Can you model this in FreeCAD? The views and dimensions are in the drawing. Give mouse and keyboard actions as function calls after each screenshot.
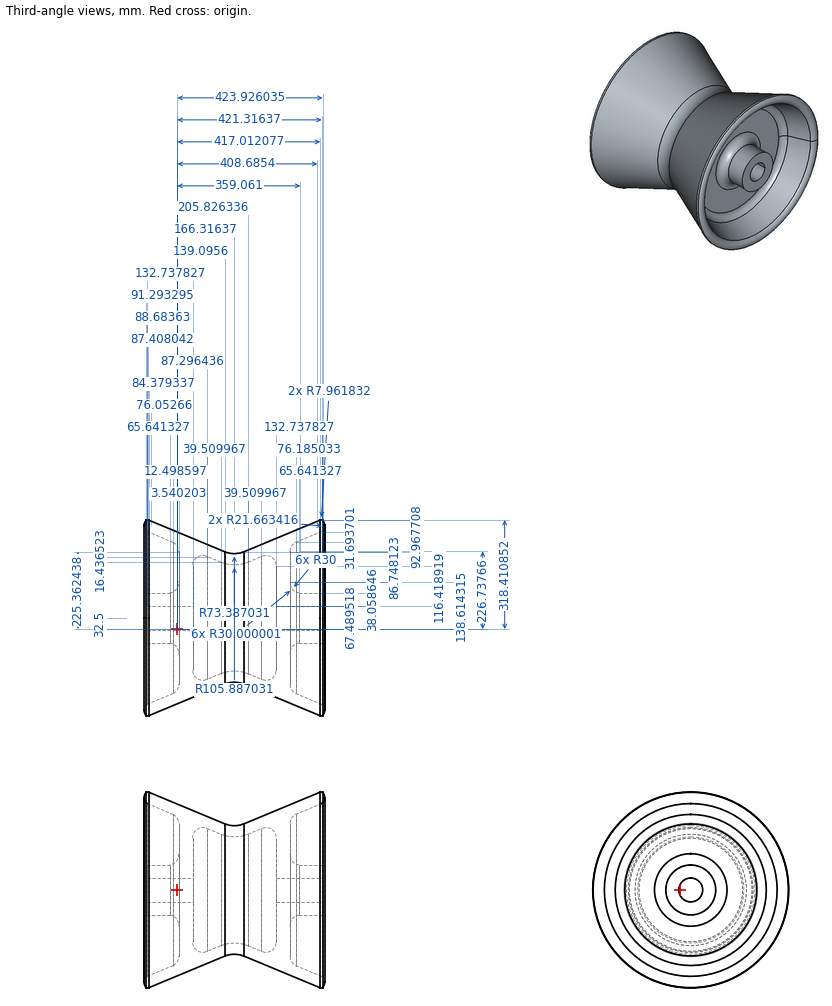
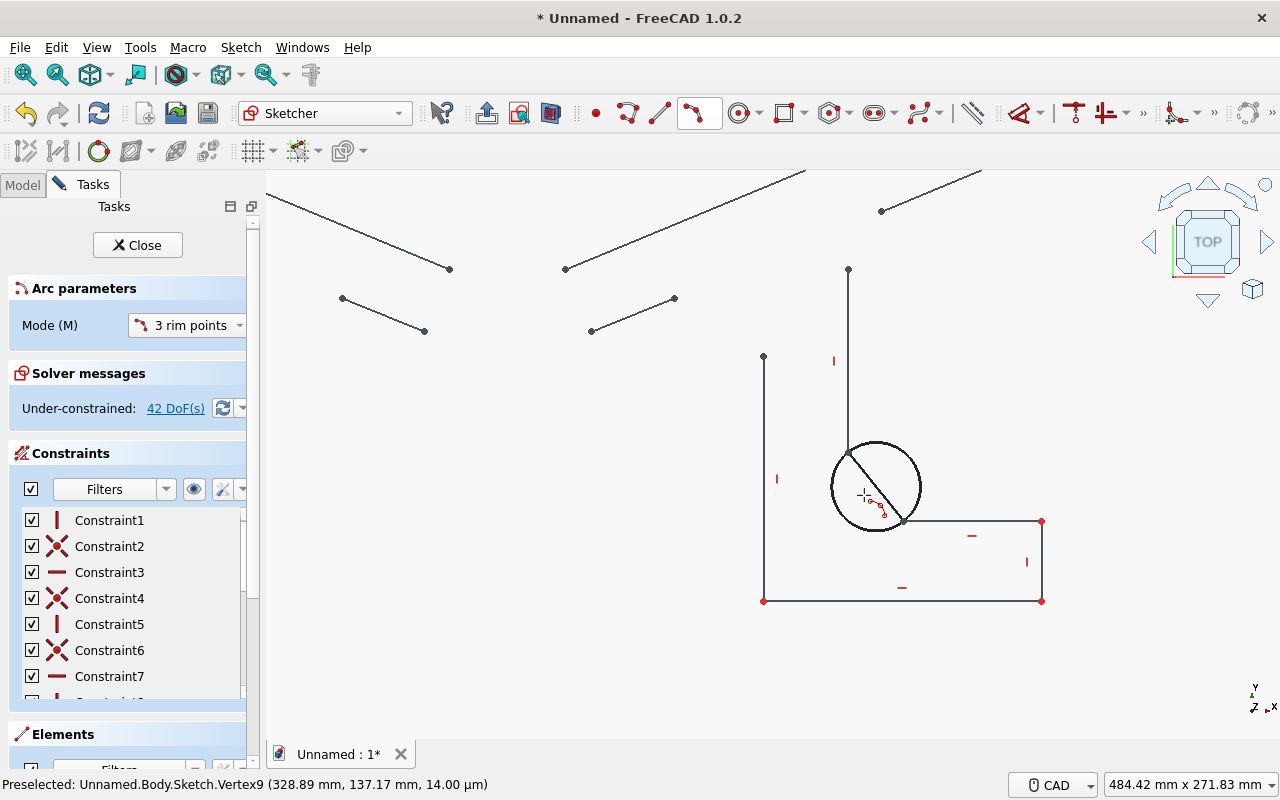
click(862, 495)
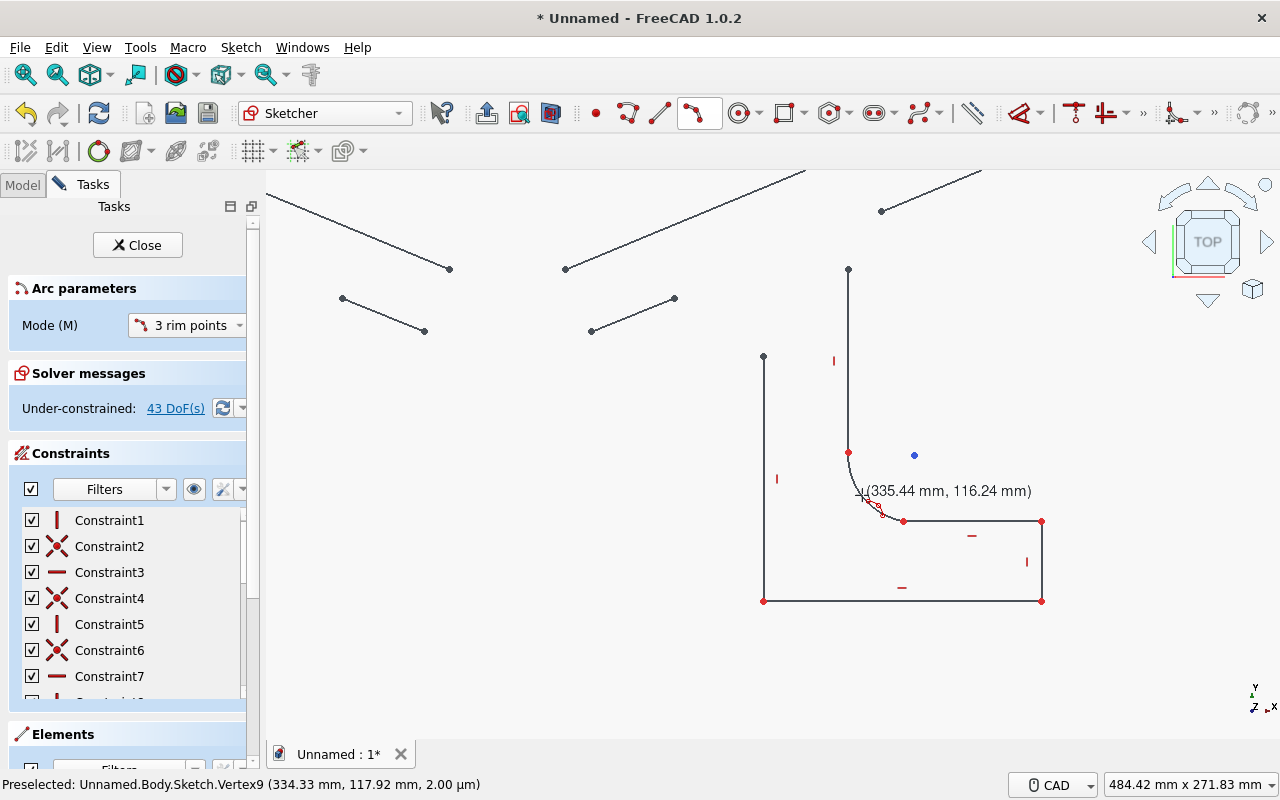
click(848, 270)
click(882, 212)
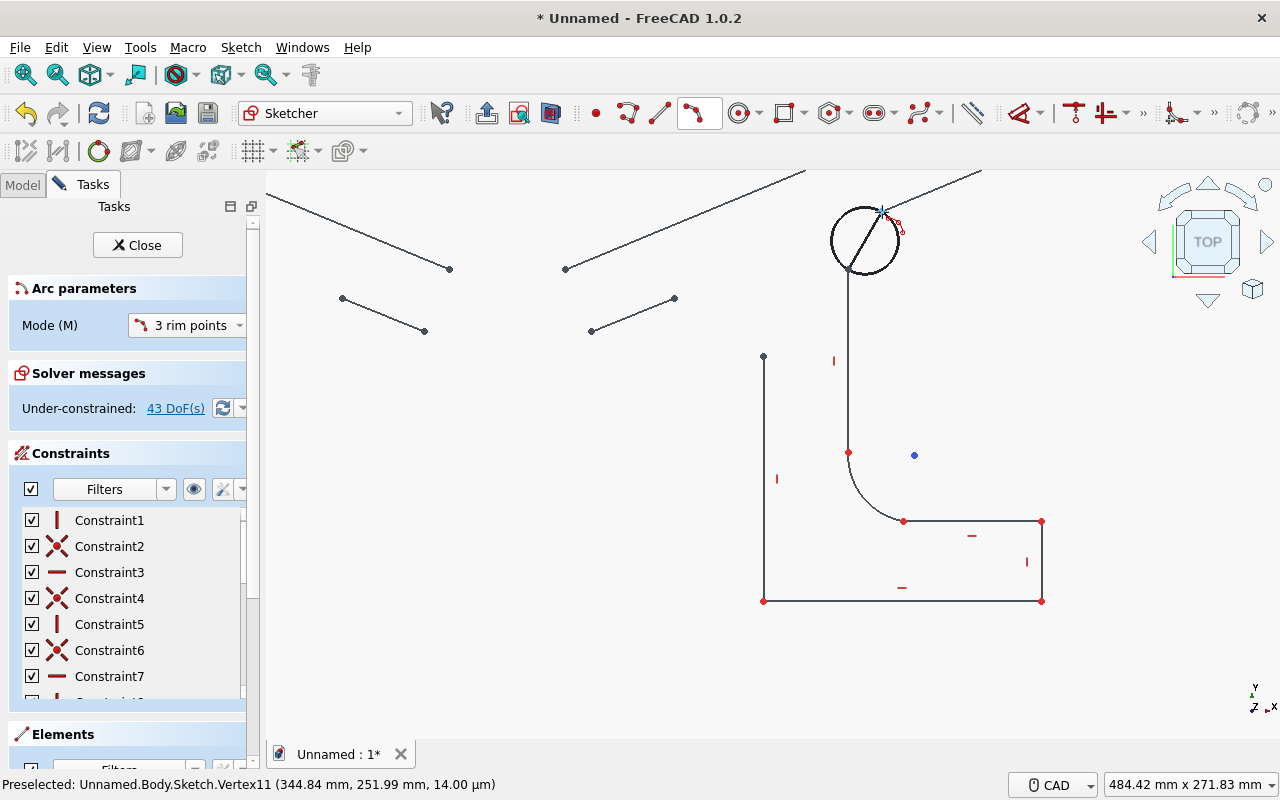
scroll(857, 233, up, 3)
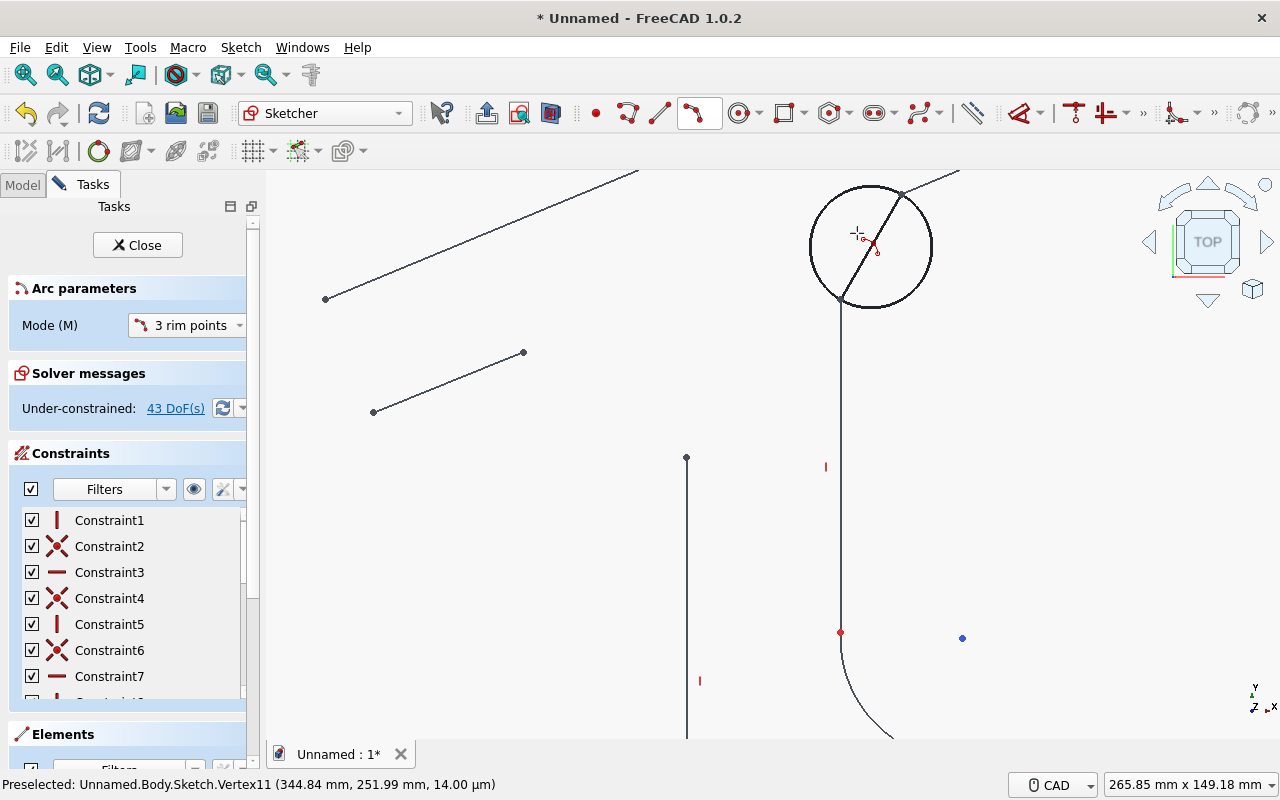
click(857, 234)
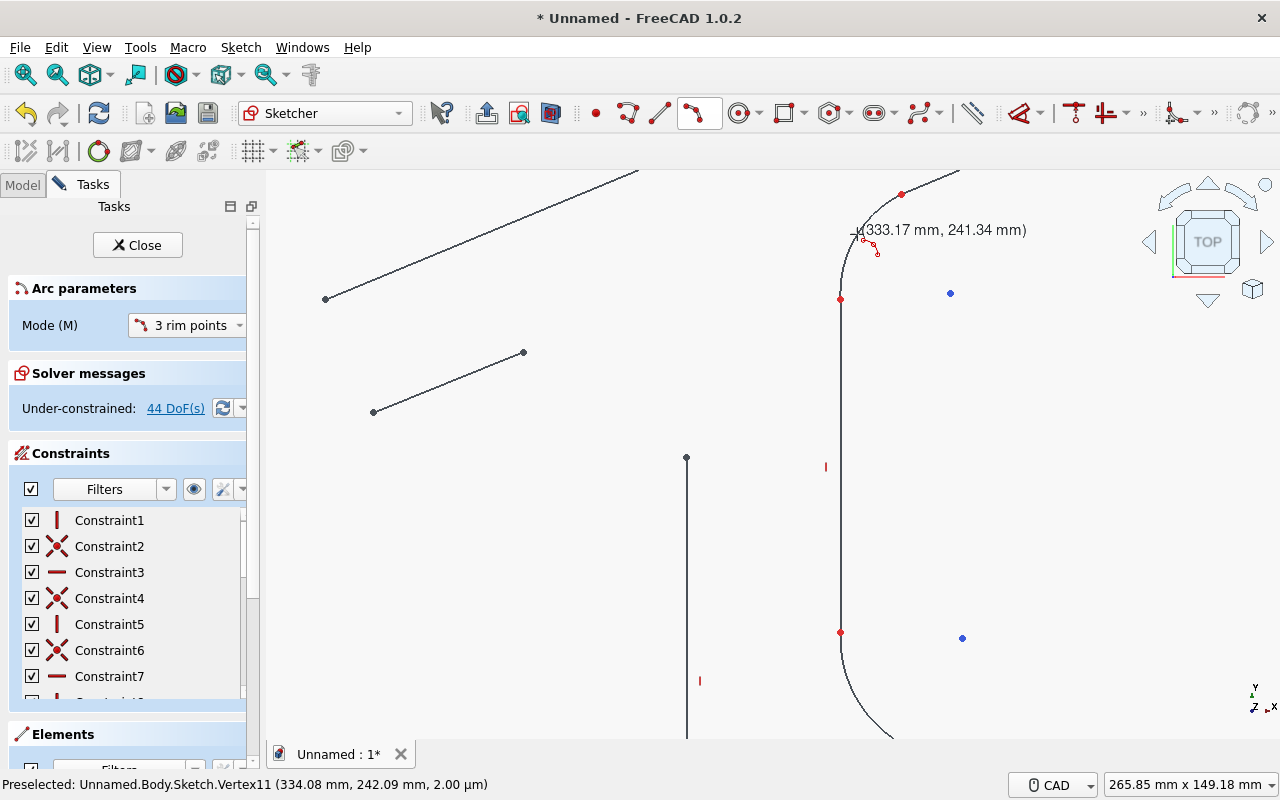
scroll(863, 424, down, 7)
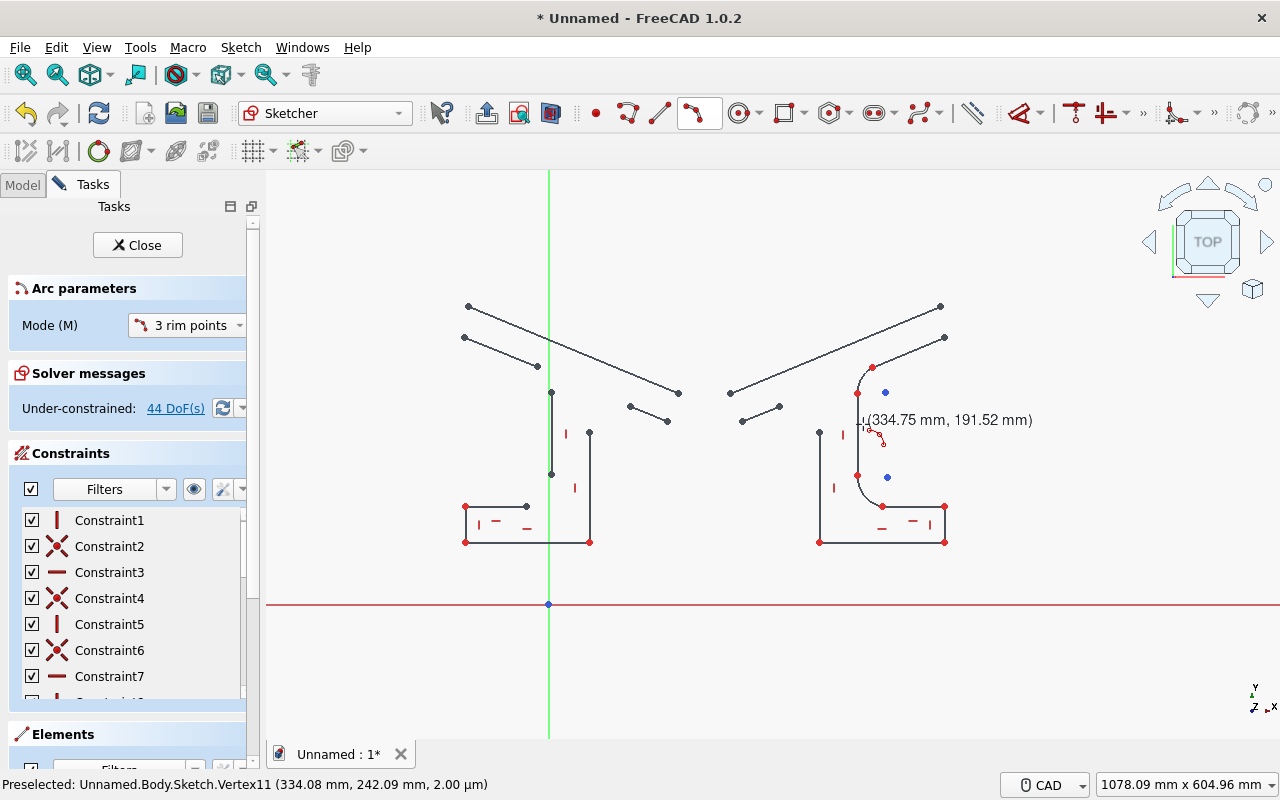
click(945, 338)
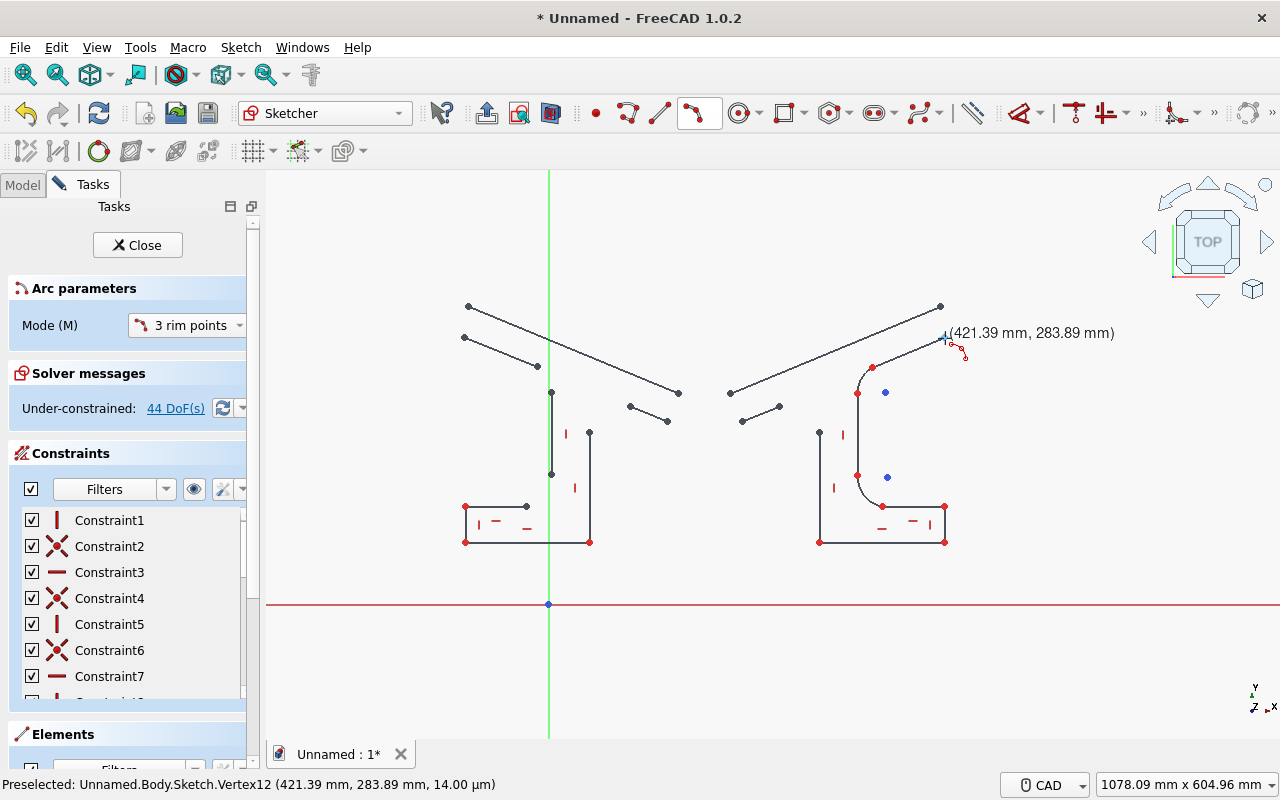
scroll(947, 306, up, 5)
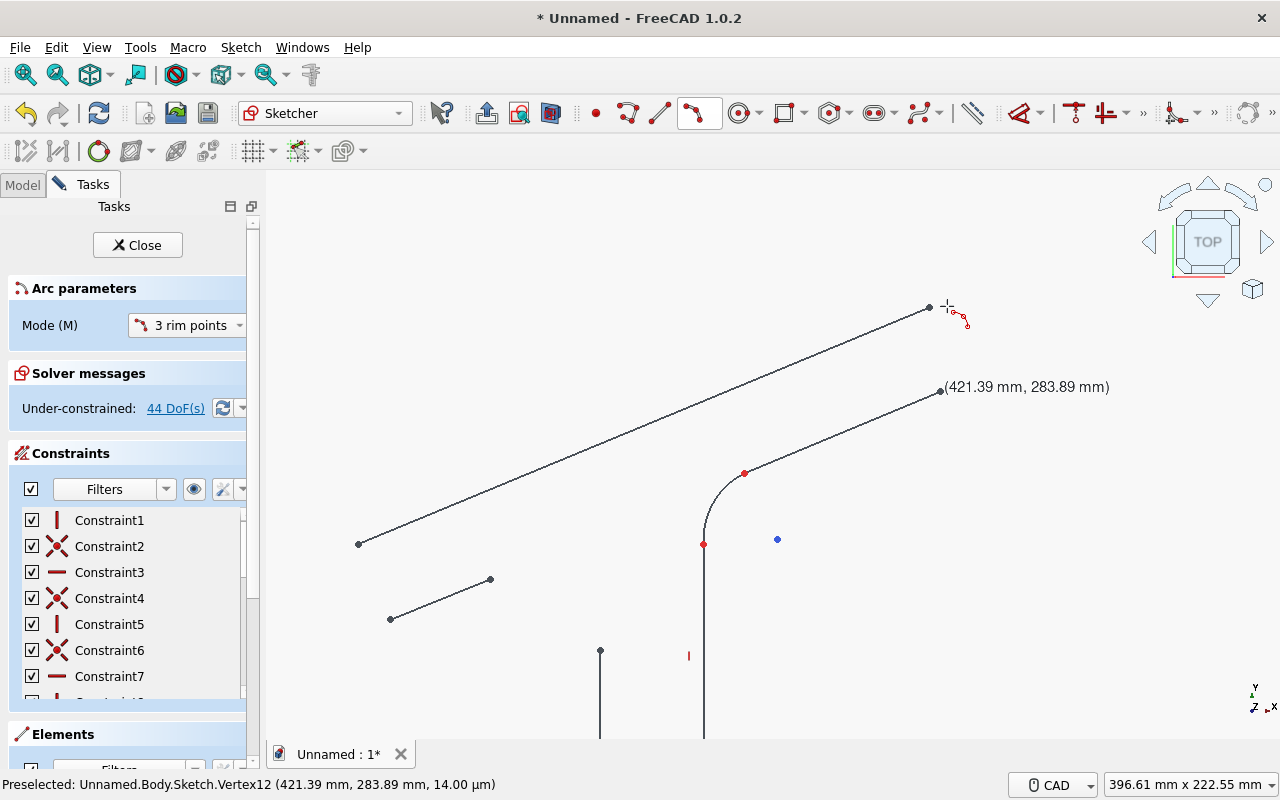
click(947, 305)
click(963, 348)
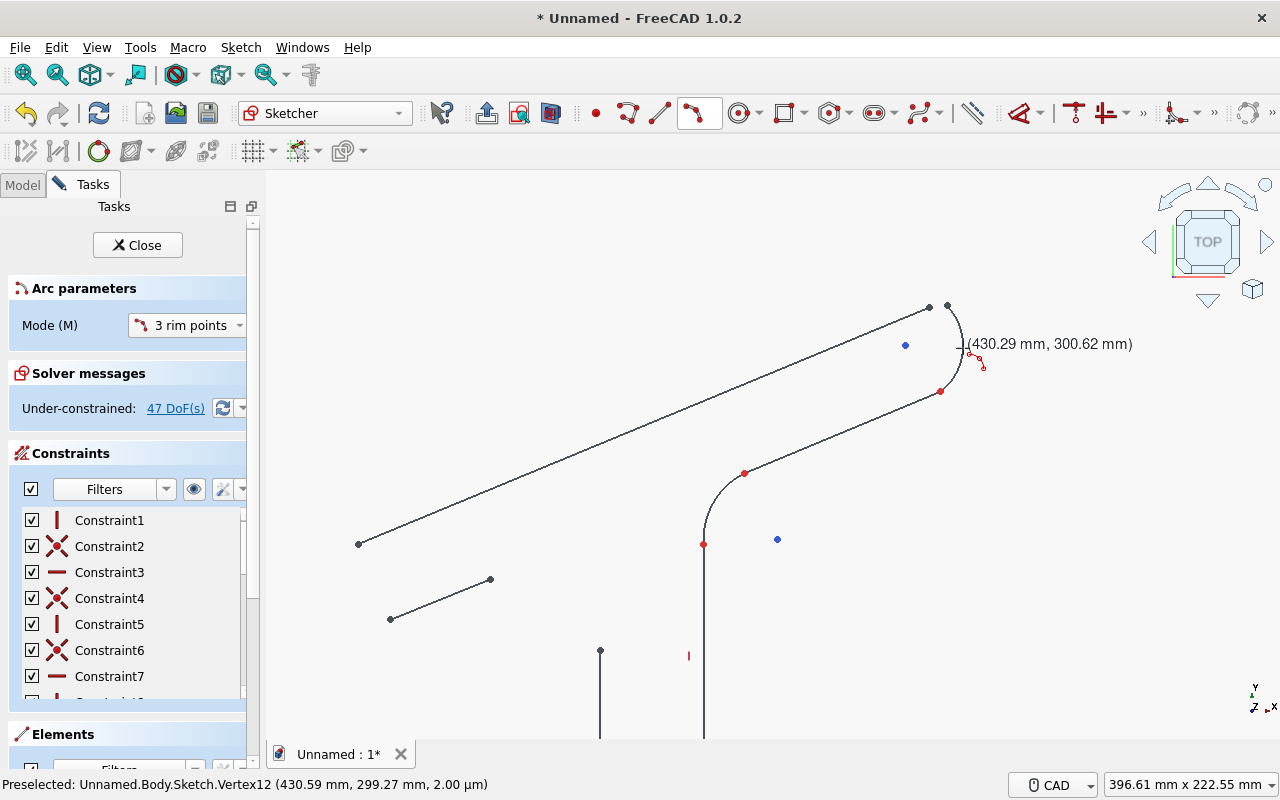
click(947, 306)
click(929, 308)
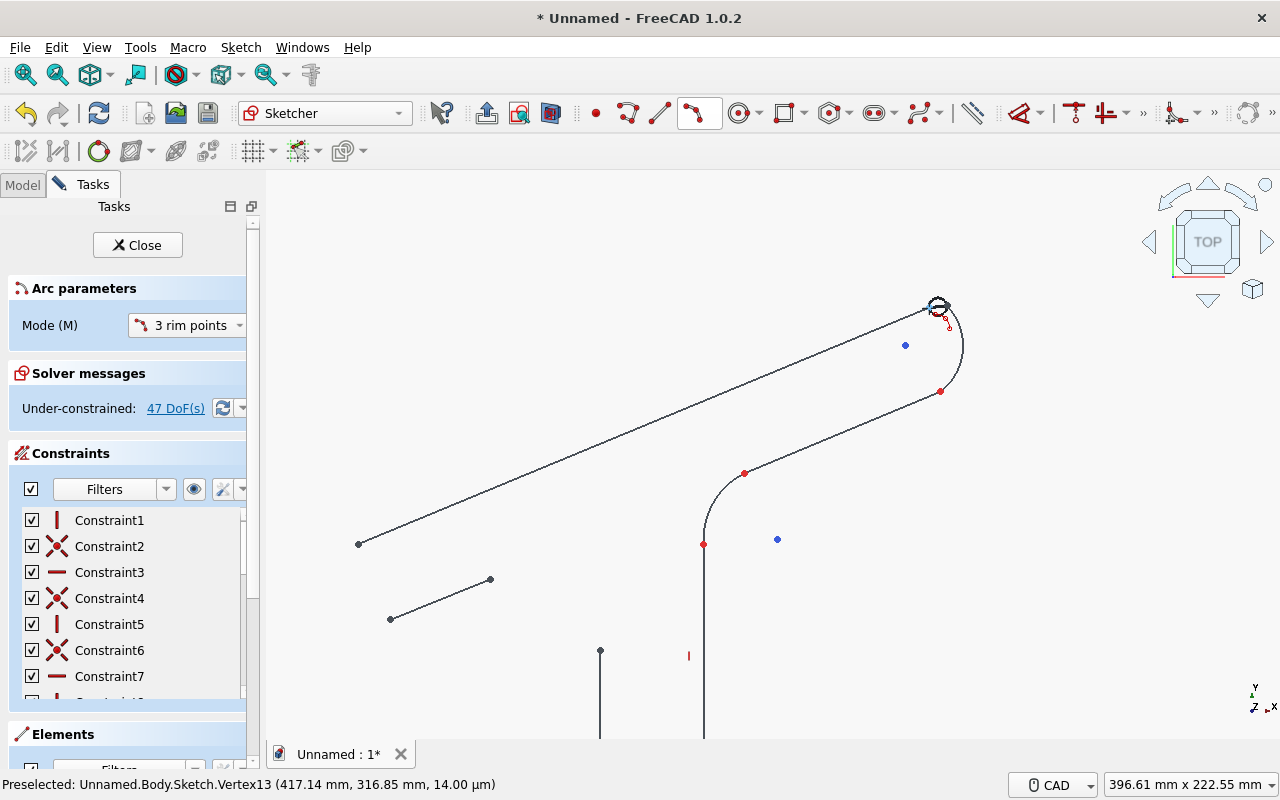
scroll(938, 302, up, 11)